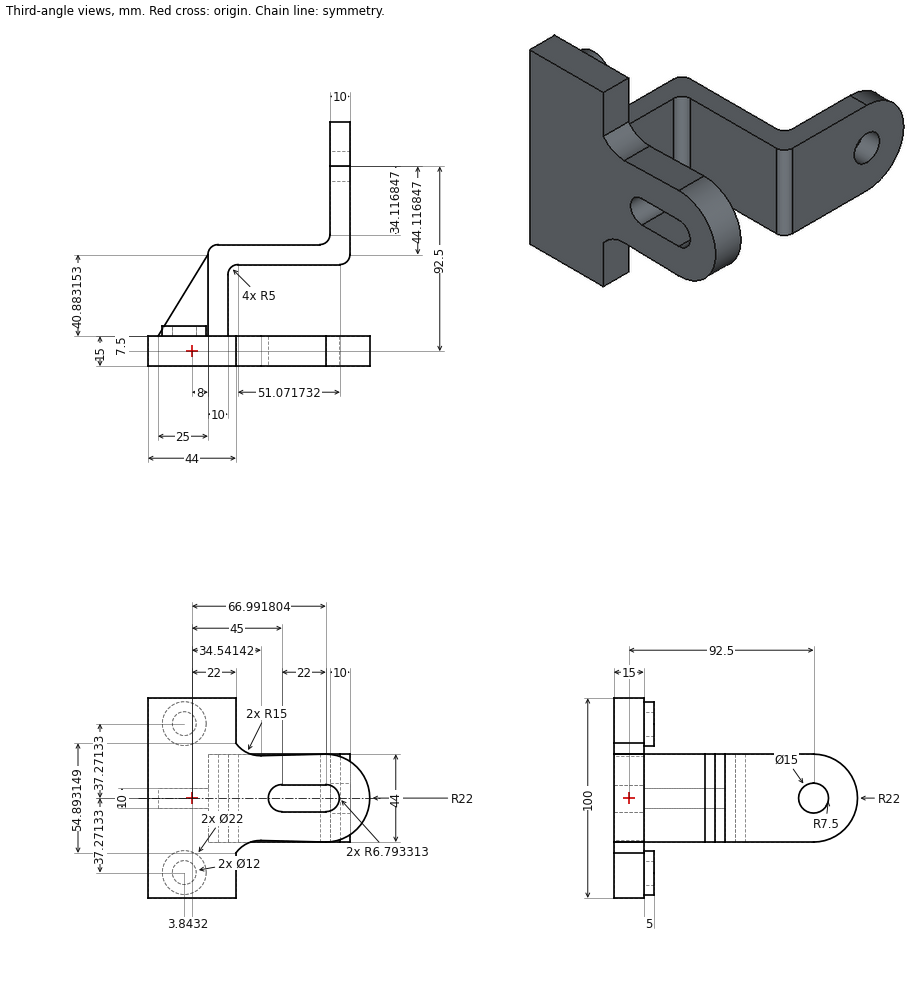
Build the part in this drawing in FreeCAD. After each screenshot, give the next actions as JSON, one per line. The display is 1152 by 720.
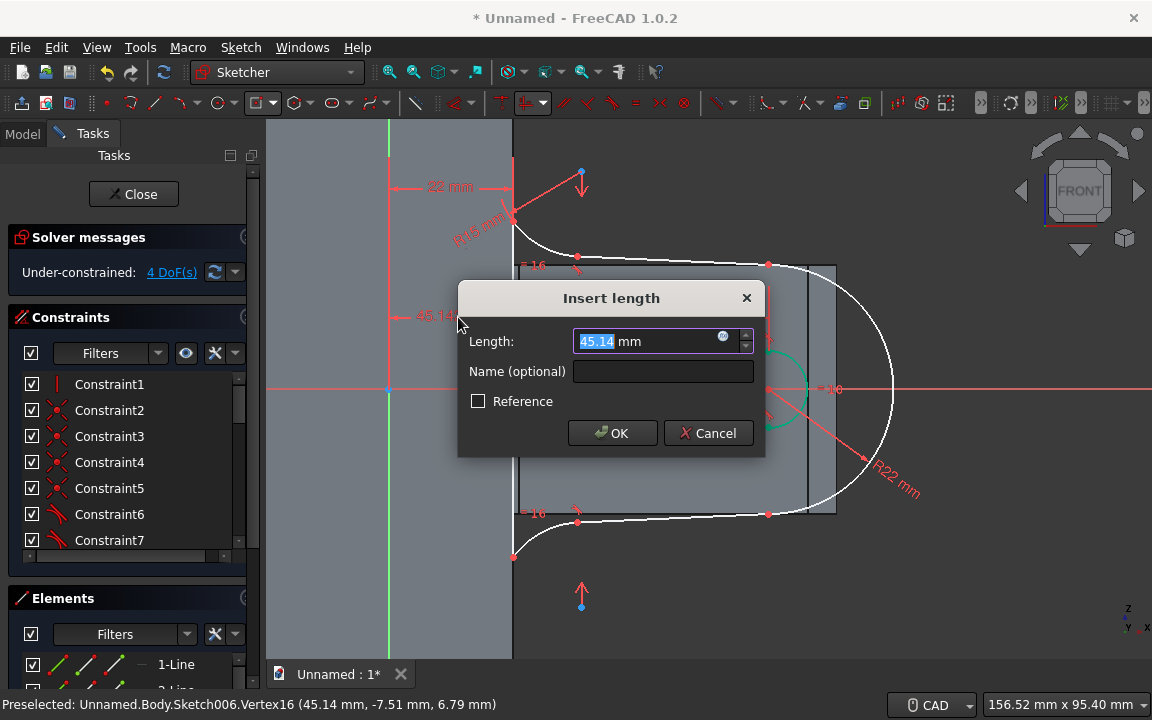
{"action": "type", "text": "45"}
{"action": "key", "text": "Return"}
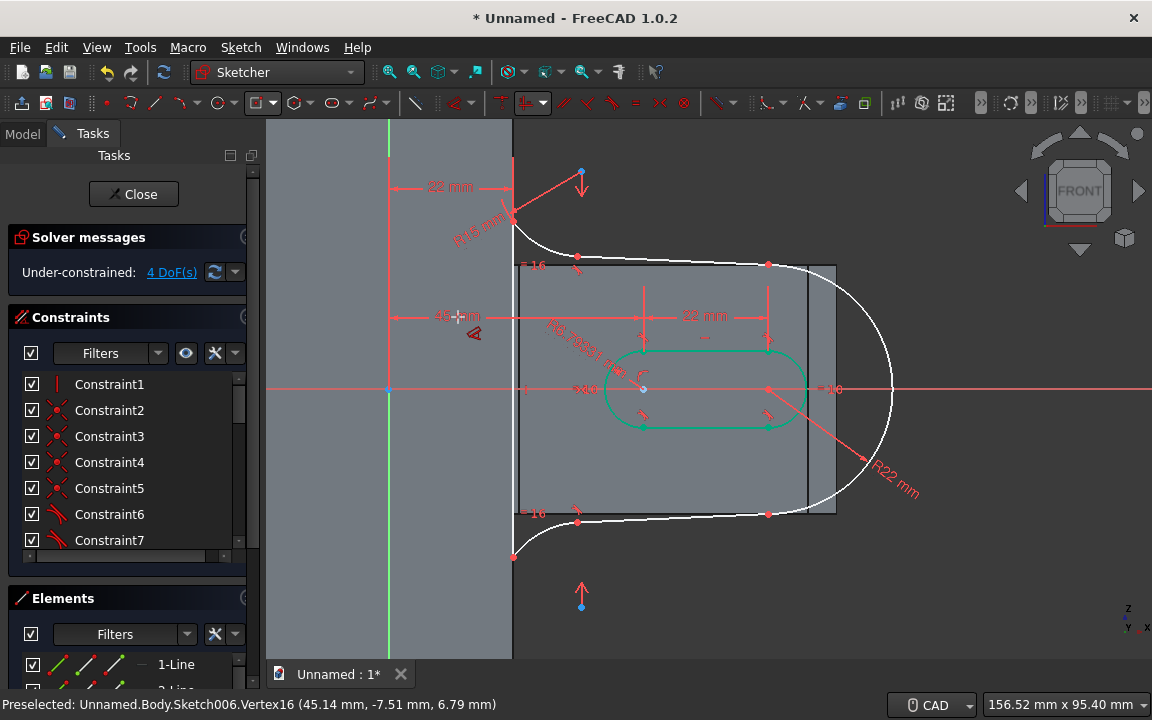
{"action": "left_click", "coordinate": [513, 322]}
{"action": "left_click", "coordinate": [479, 467]}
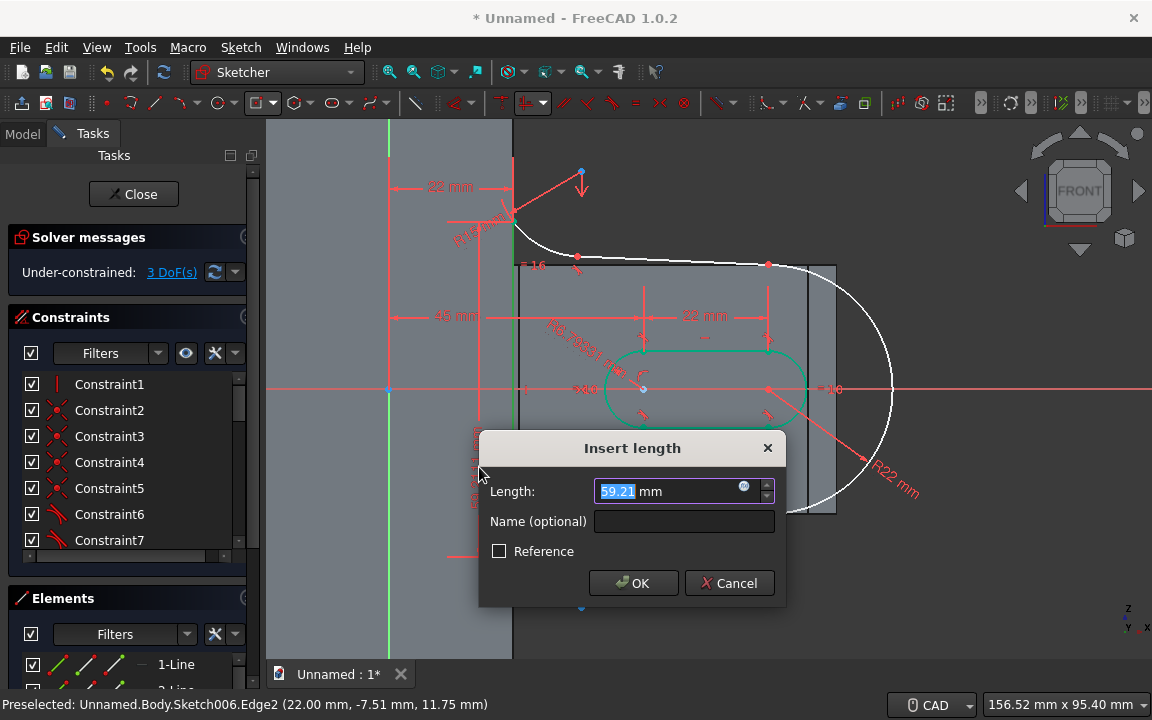
{"action": "type", "text": "54.893149"}
{"action": "key", "text": "Return"}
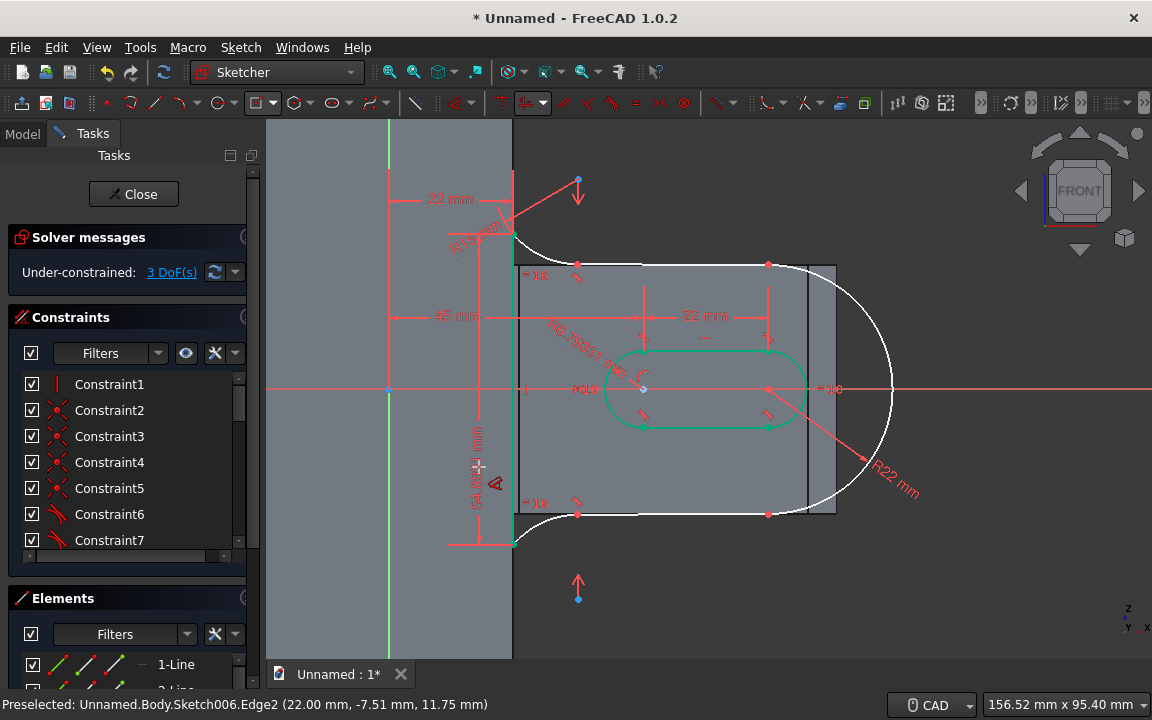
{"action": "left_click", "coordinate": [578, 264]}
{"action": "left_click", "coordinate": [550, 230]}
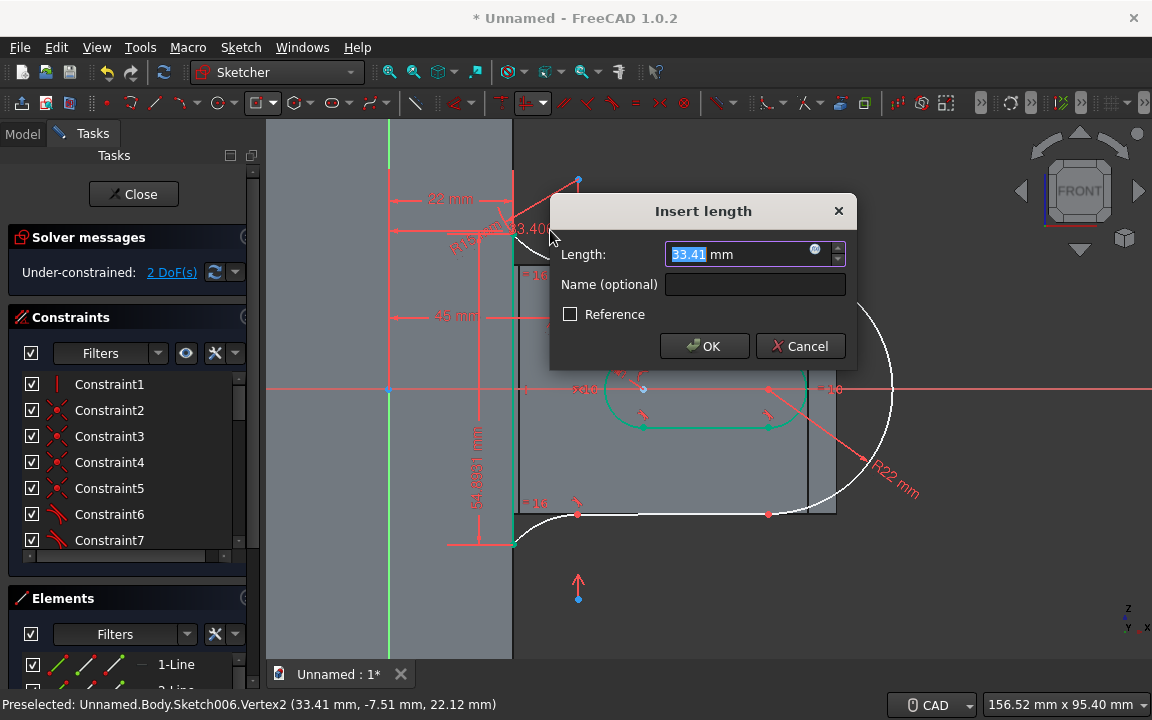
{"action": "type", "text": "34.54142"}
{"action": "key", "text": "Return"}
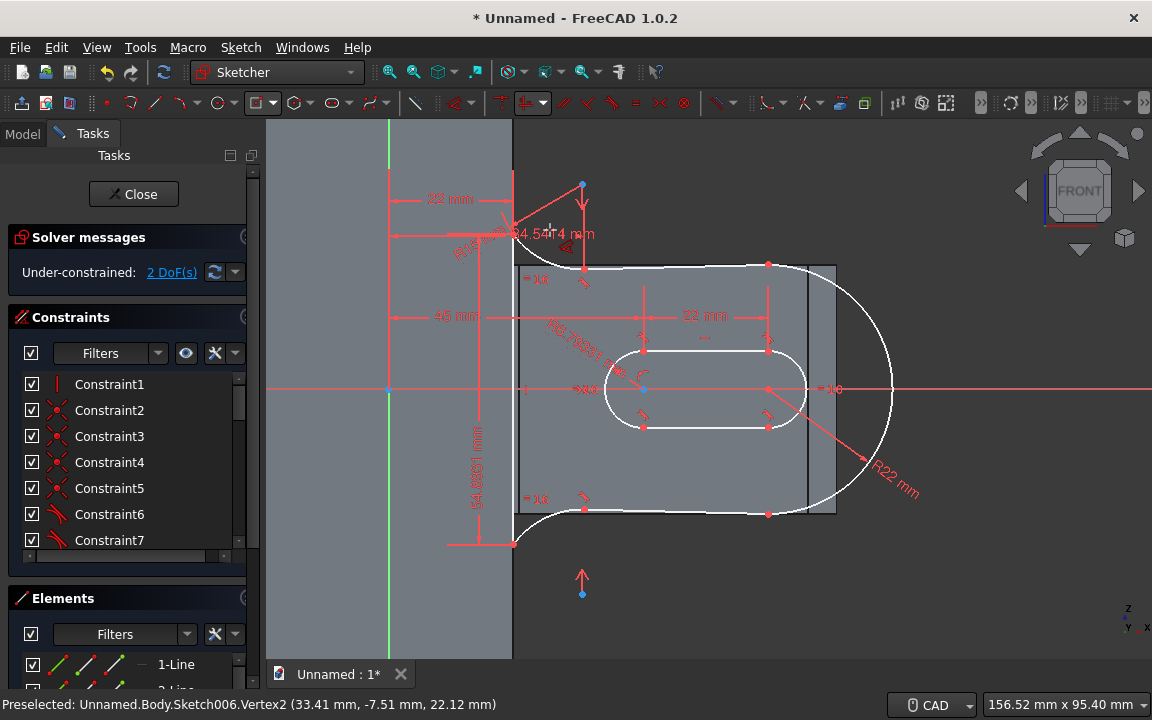
{"action": "left_click", "coordinate": [768, 265]}
{"action": "left_click", "coordinate": [666, 231]}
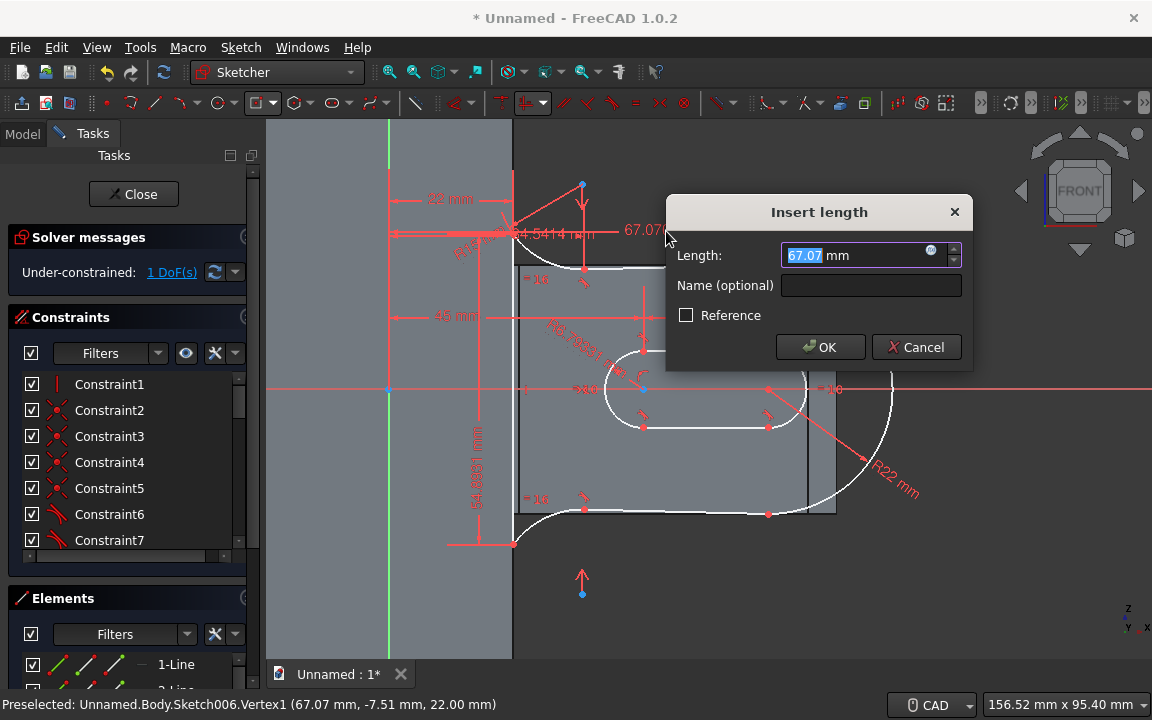
{"action": "type", "text": "66.991804"}
{"action": "key", "text": "Return"}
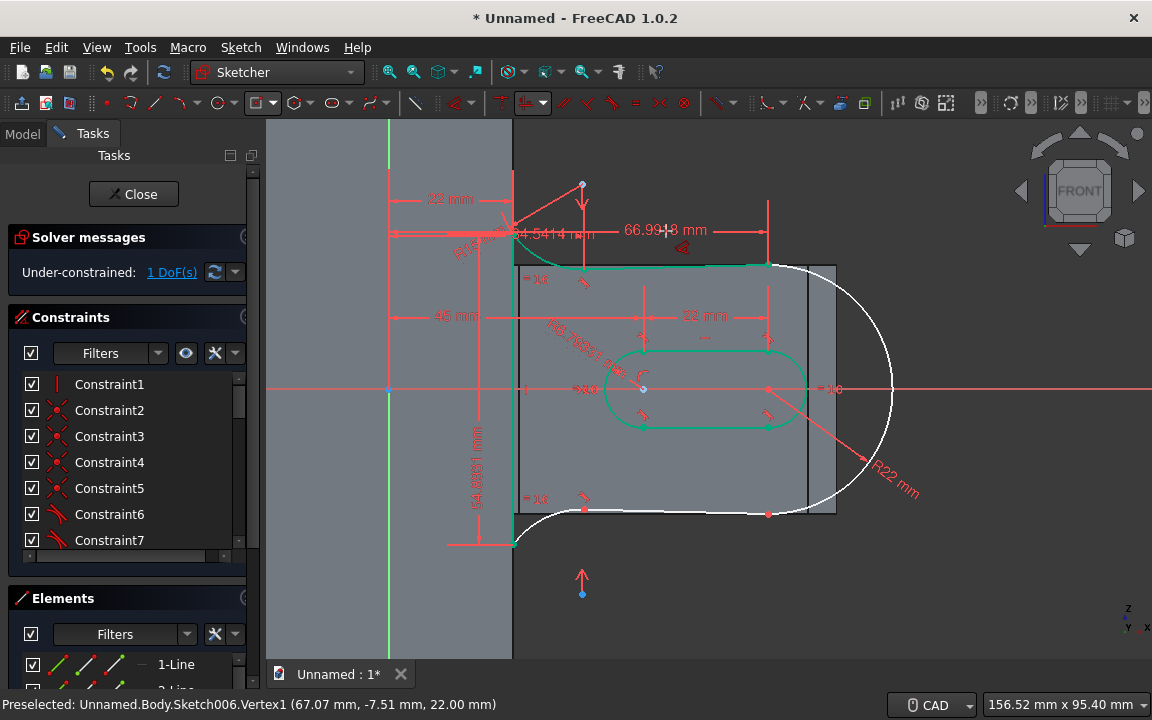
{"action": "left_click", "coordinate": [768, 514]}
{"action": "left_click", "coordinate": [579, 548]}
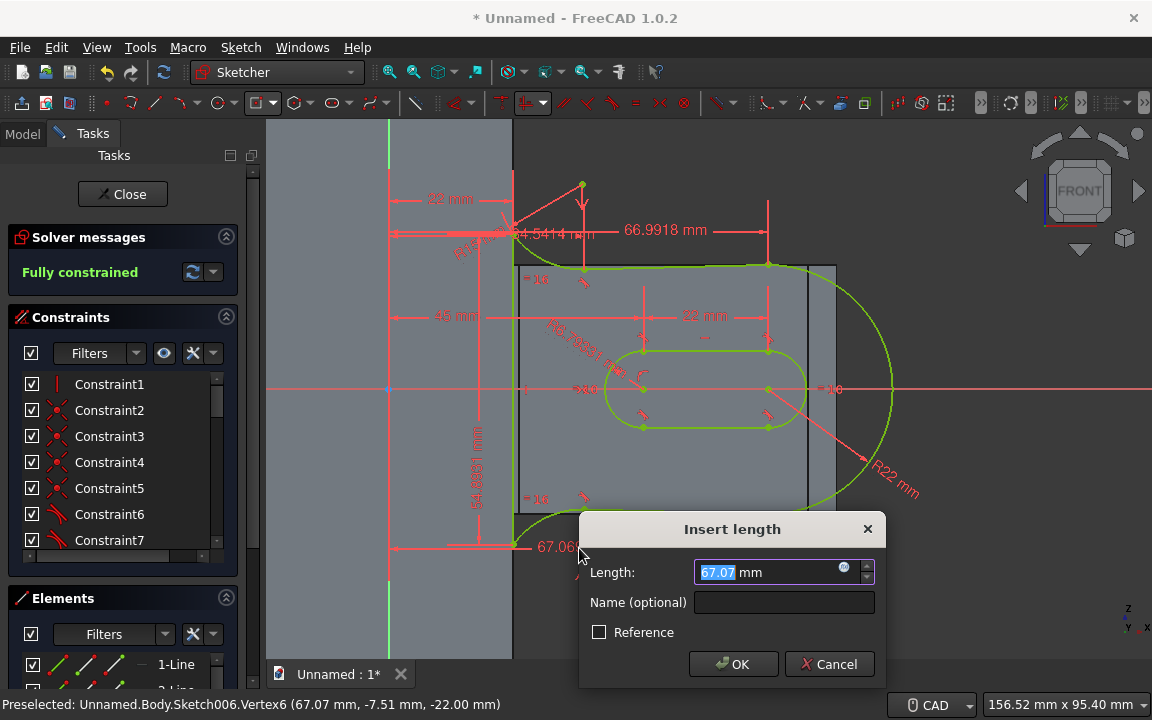
{"action": "type", "text": "66.991804"}
{"action": "key", "text": "Return"}
{"action": "key", "text": "Escape"}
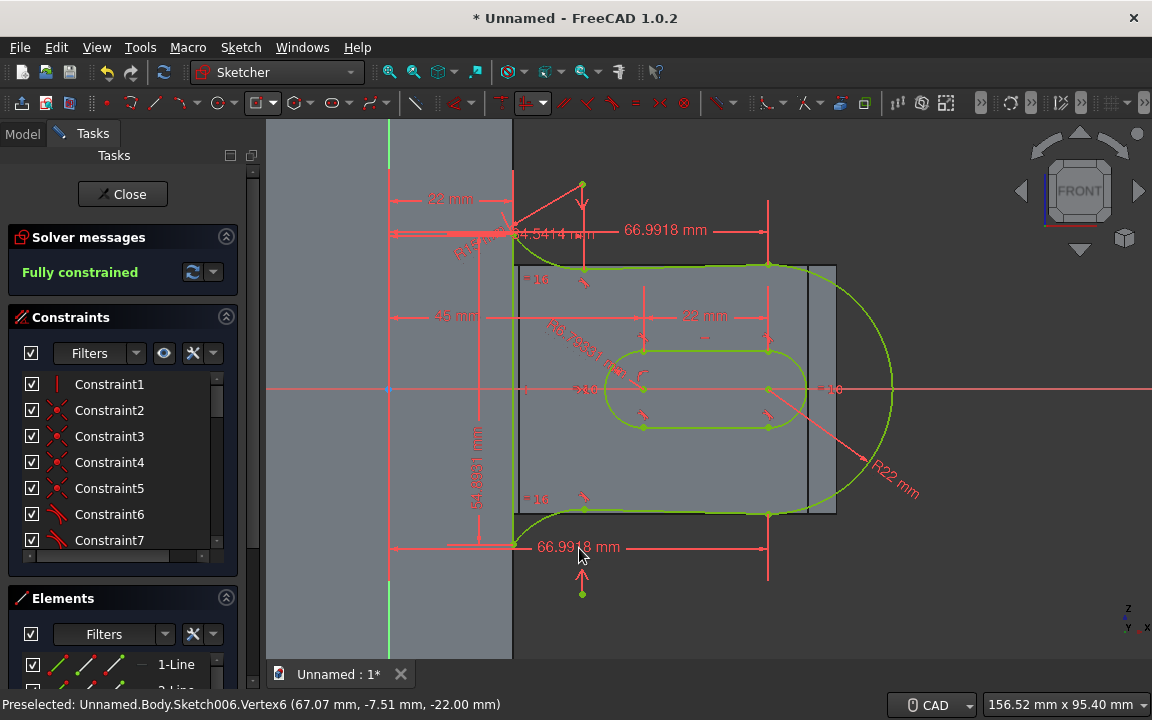
{"action": "left_click", "coordinate": [123, 194]}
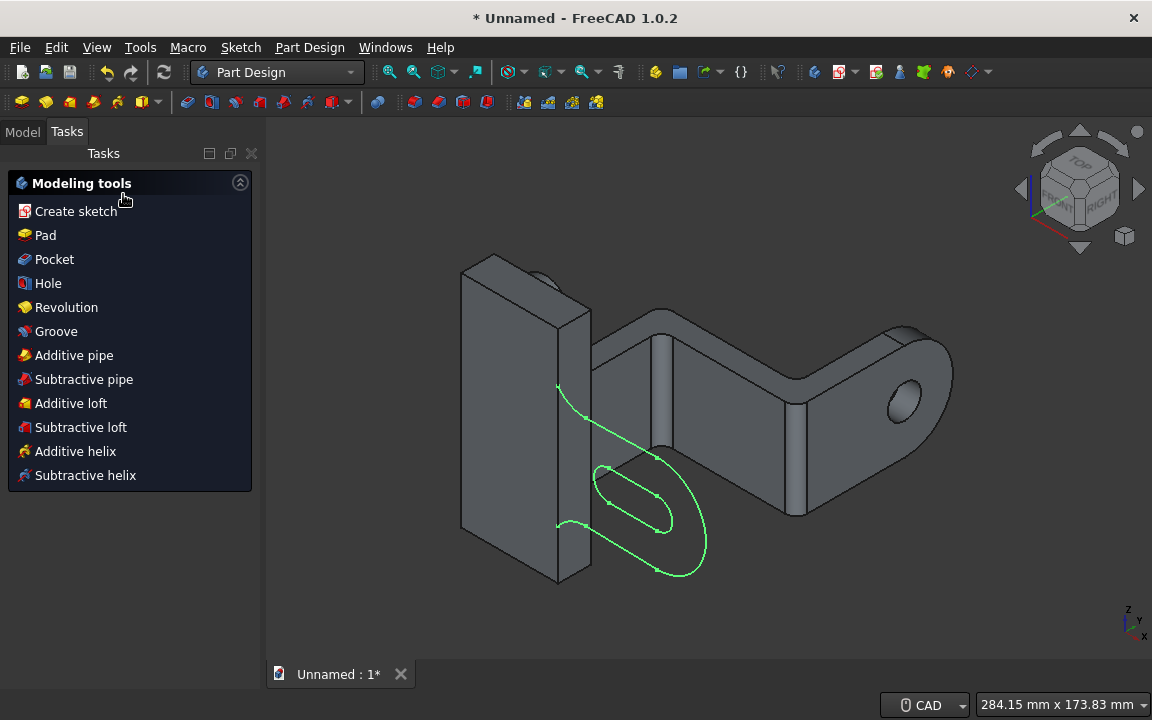
{"action": "left_click", "coordinate": [22, 102]}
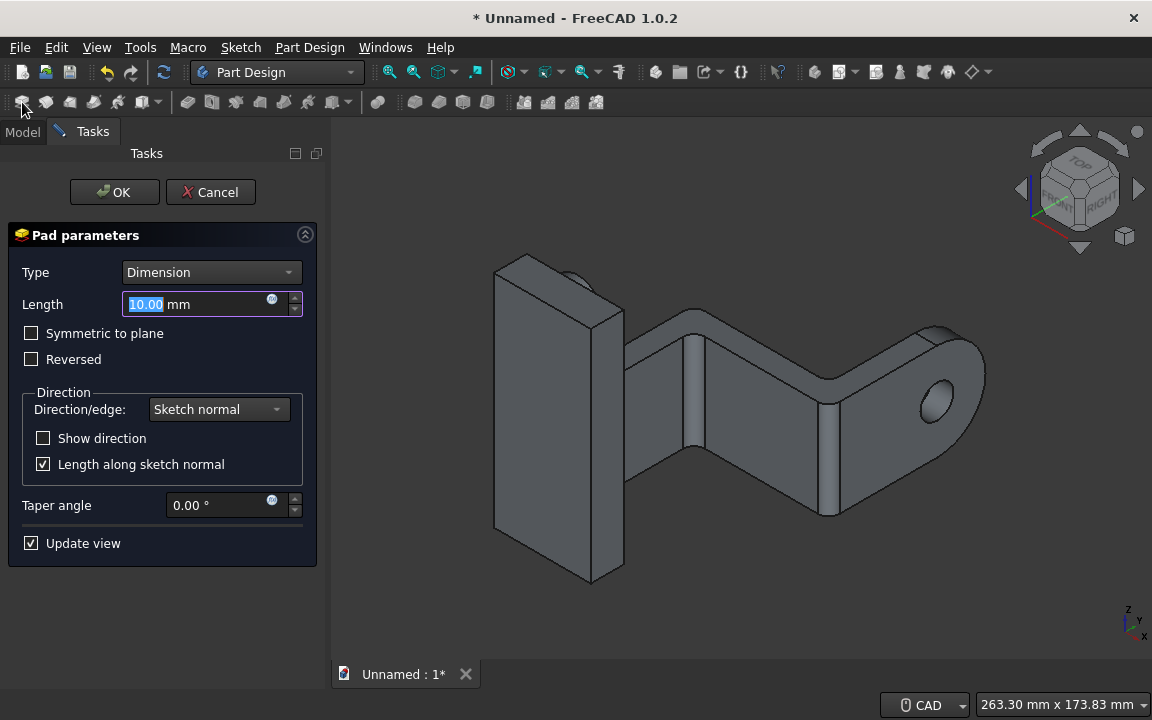
{"action": "type", "text": "15"}
{"action": "key", "text": "Tab"}